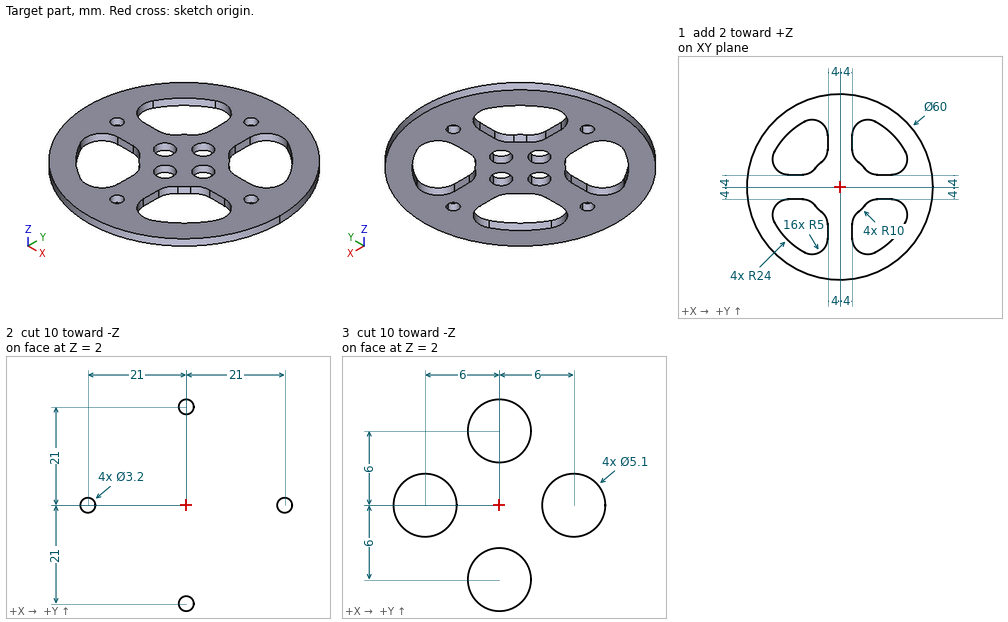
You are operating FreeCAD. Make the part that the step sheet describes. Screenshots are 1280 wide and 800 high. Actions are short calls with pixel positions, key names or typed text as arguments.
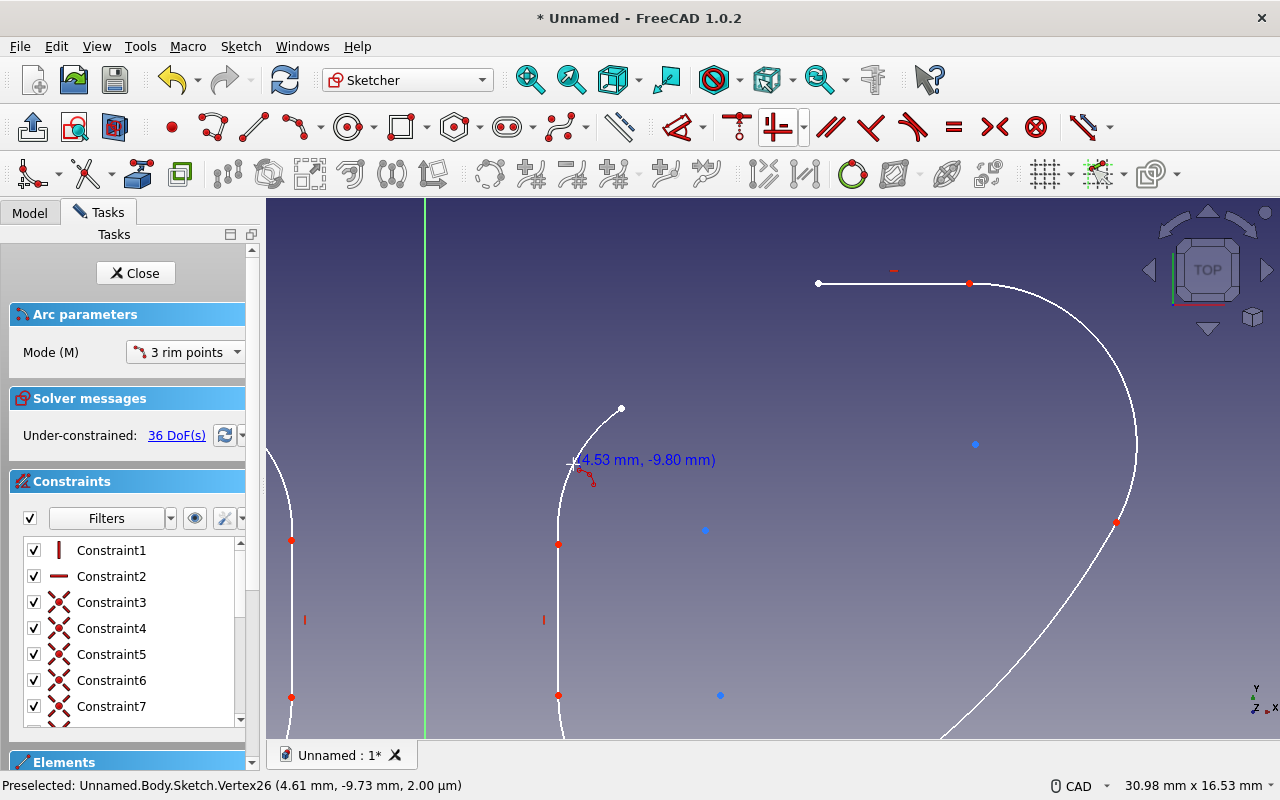
scroll(760, 533, down, 9)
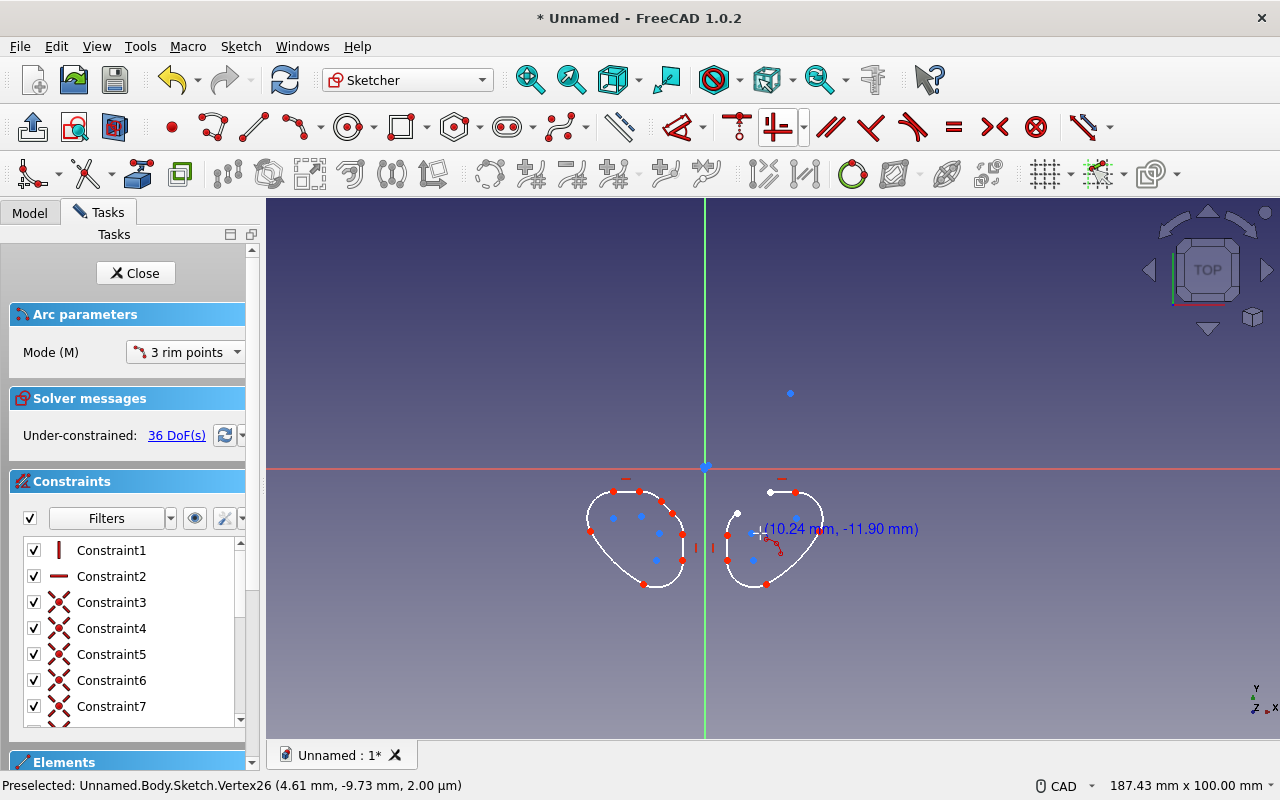
click(737, 513)
click(748, 502)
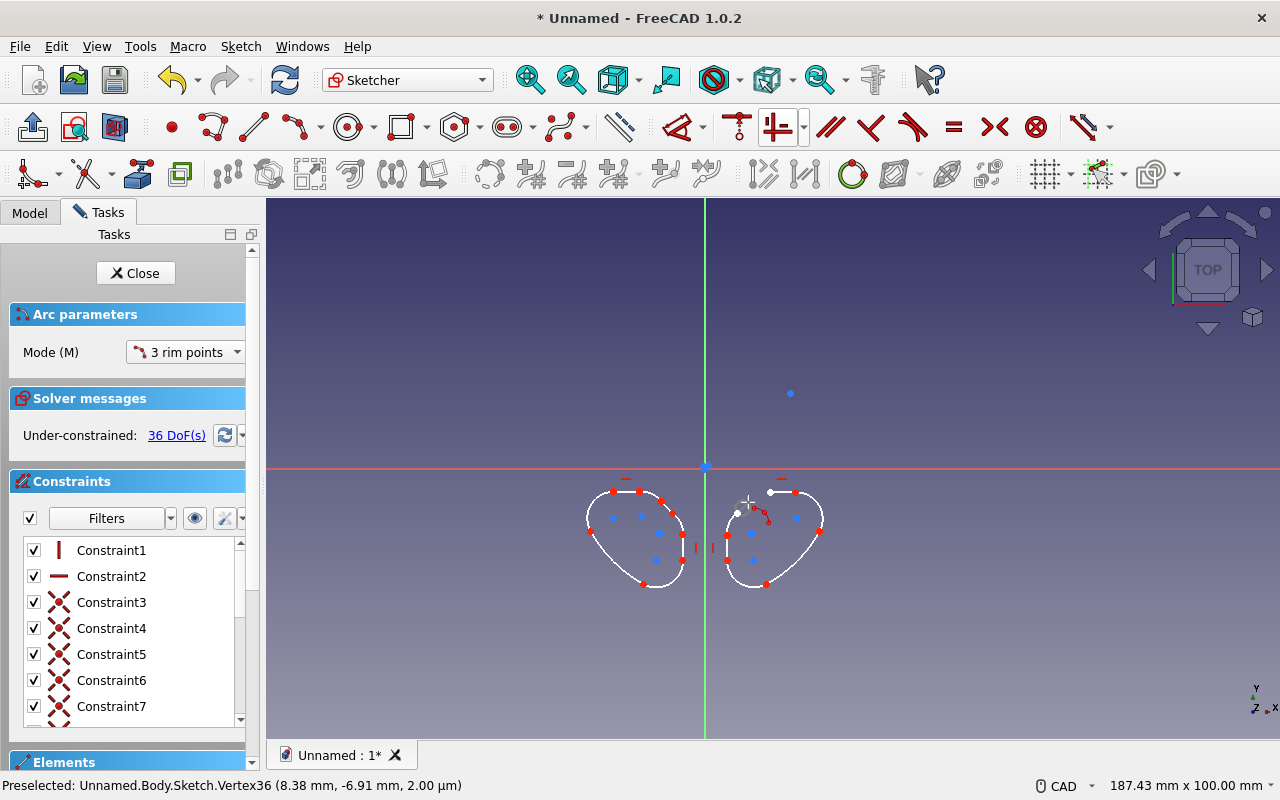
scroll(743, 508, up, 17)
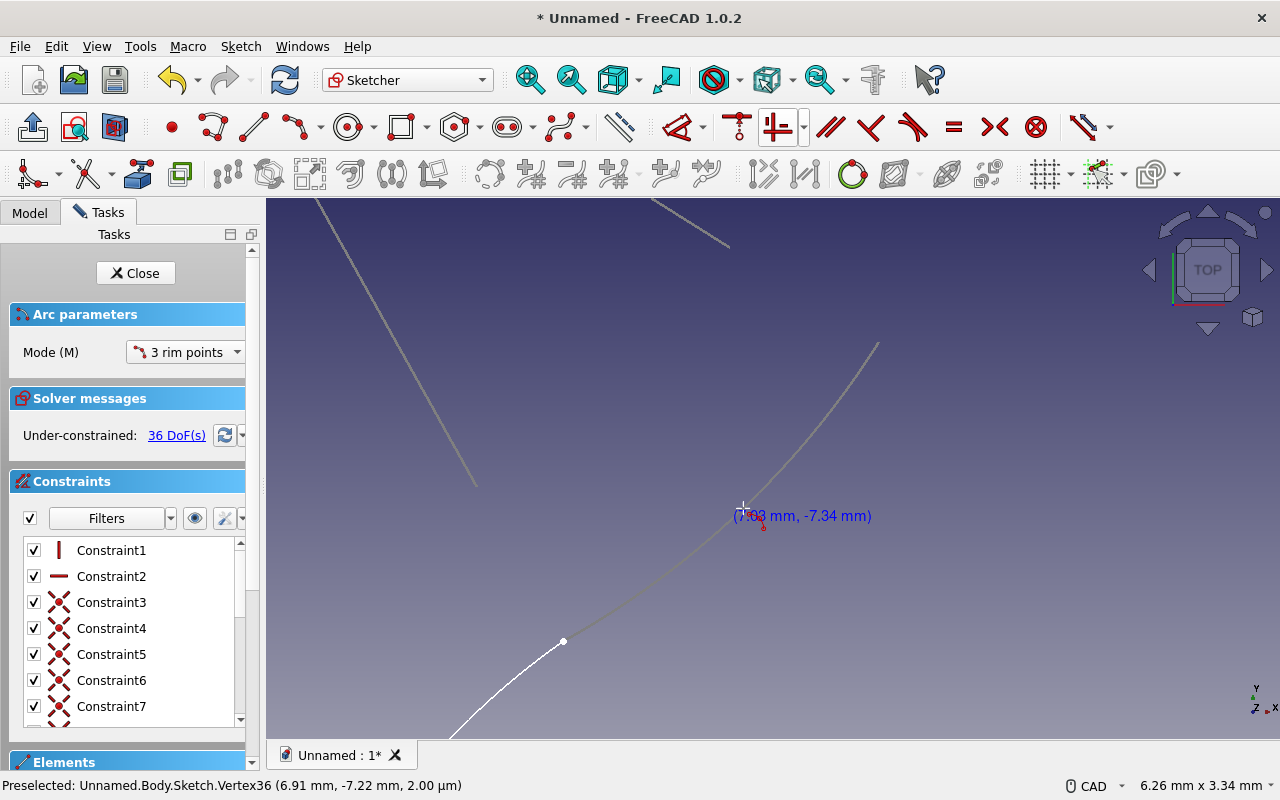
click(737, 478)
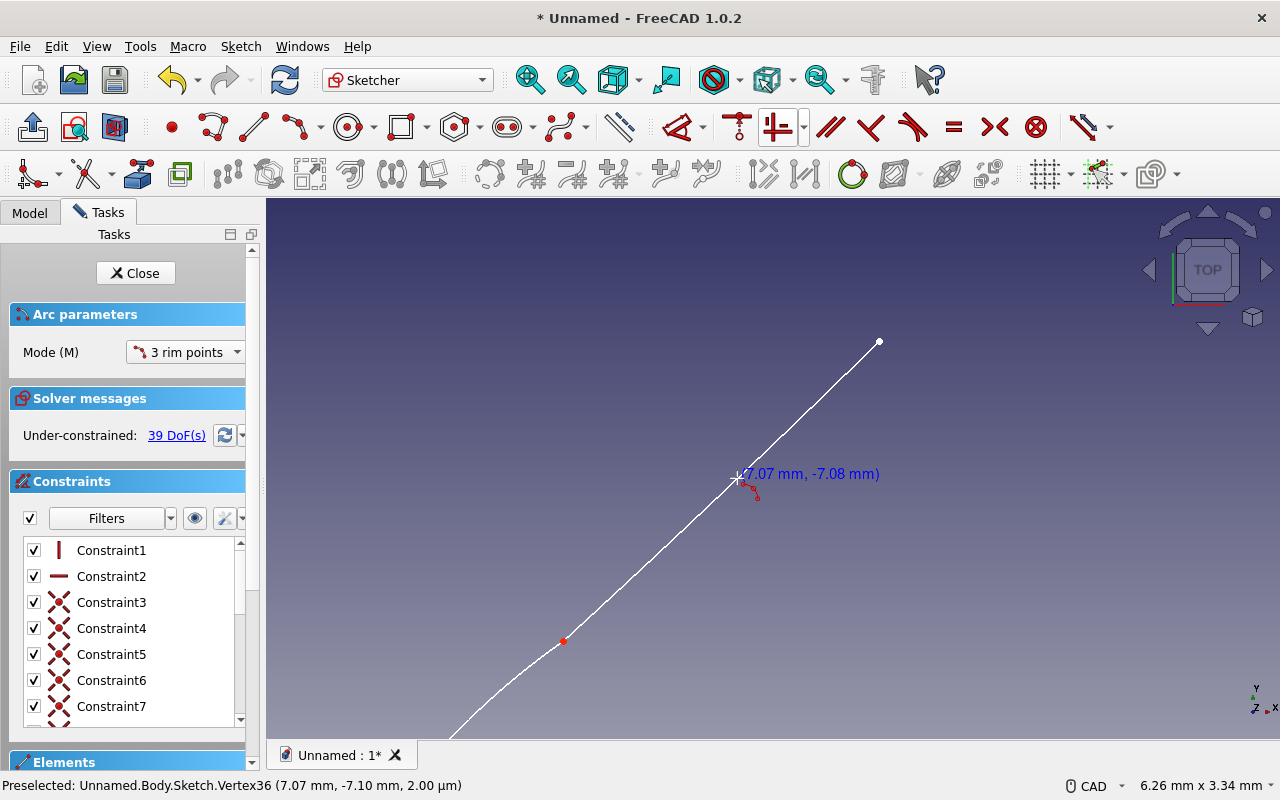
scroll(752, 517, down, 16)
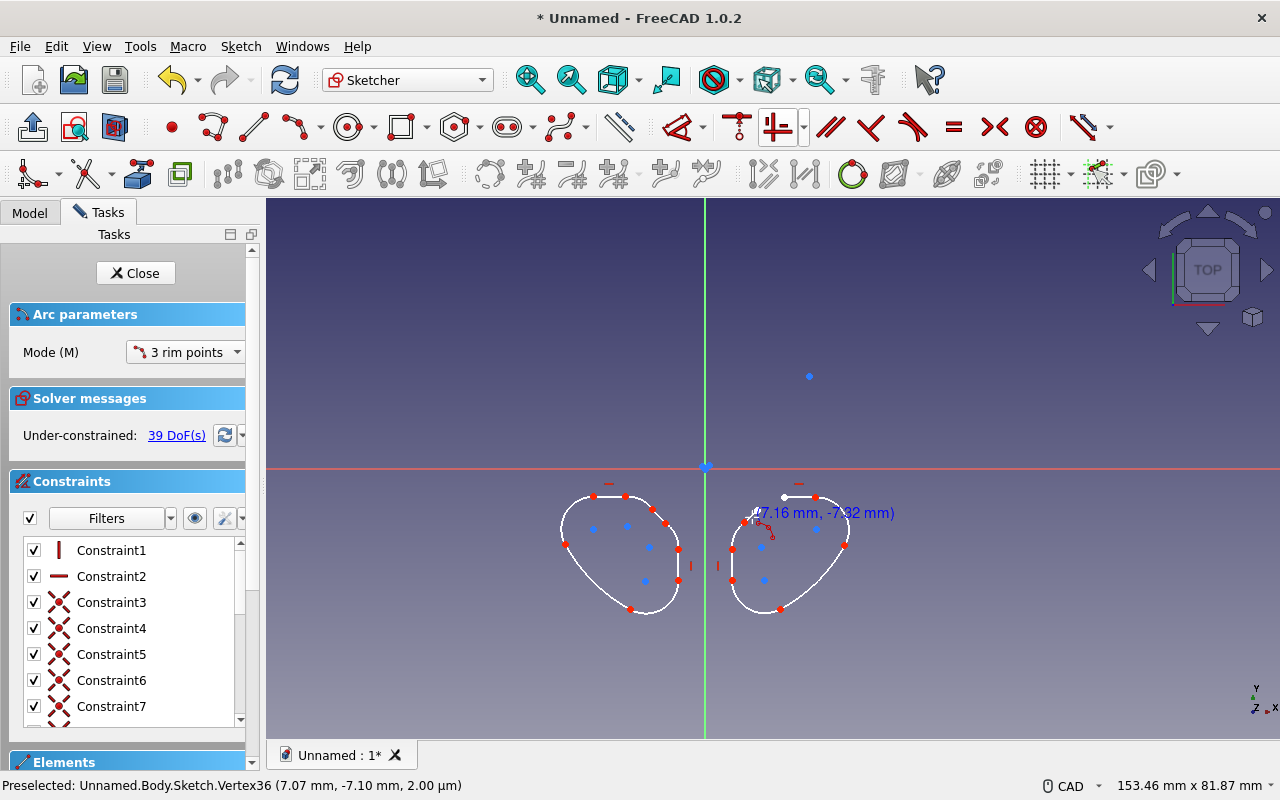
click(758, 510)
click(785, 497)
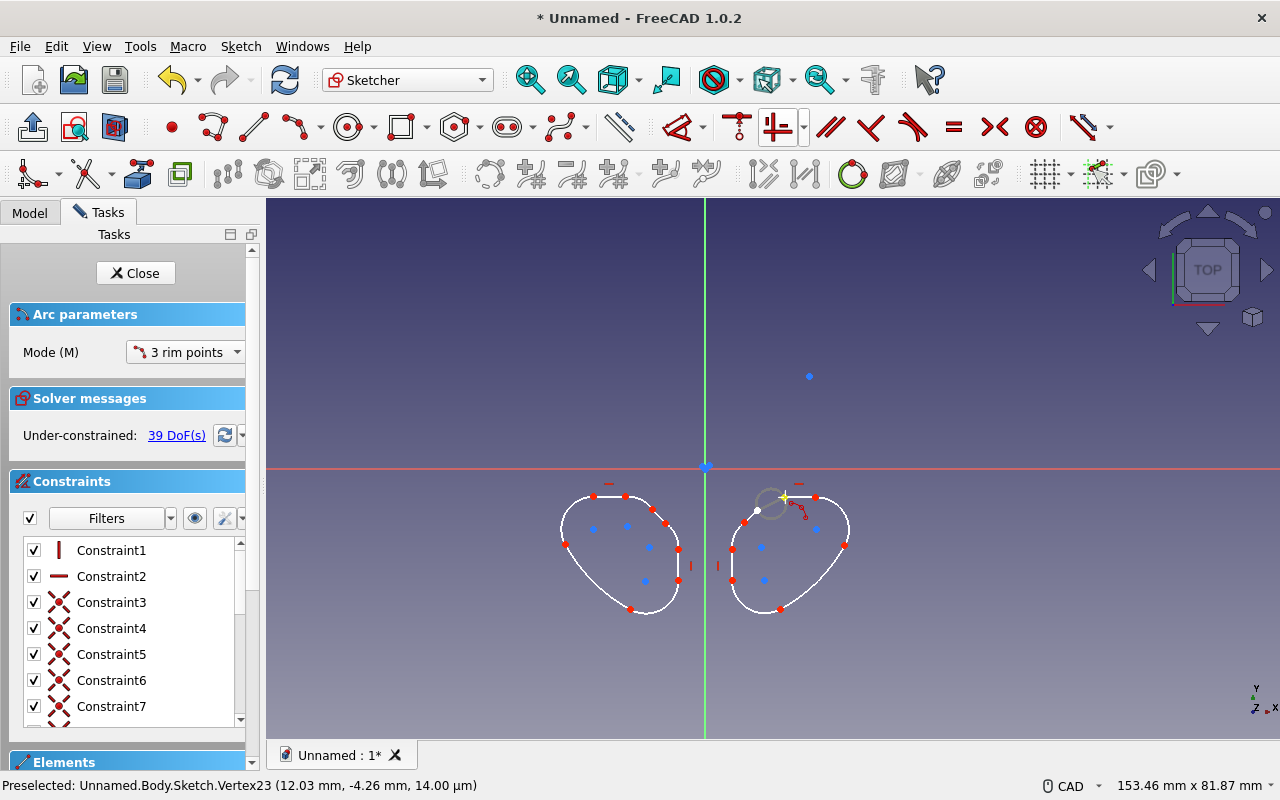
scroll(770, 499, up, 8)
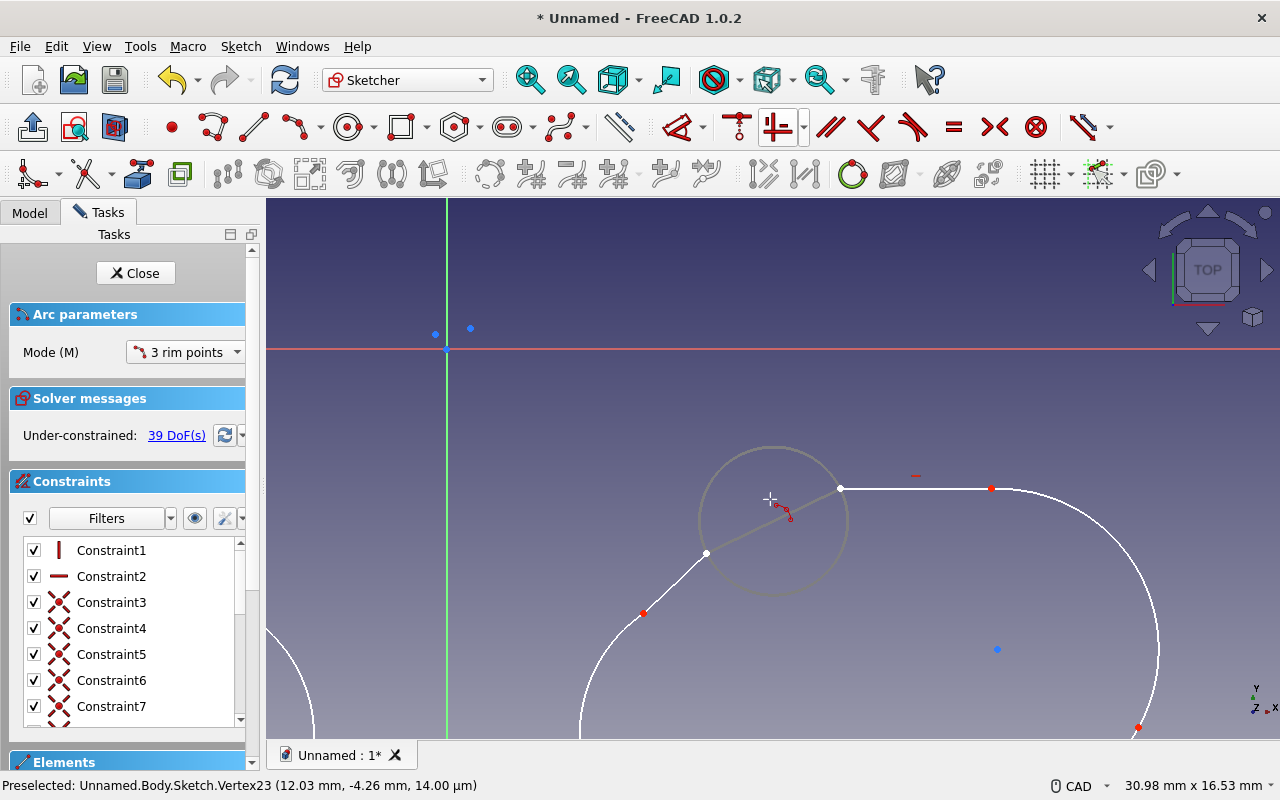
click(766, 498)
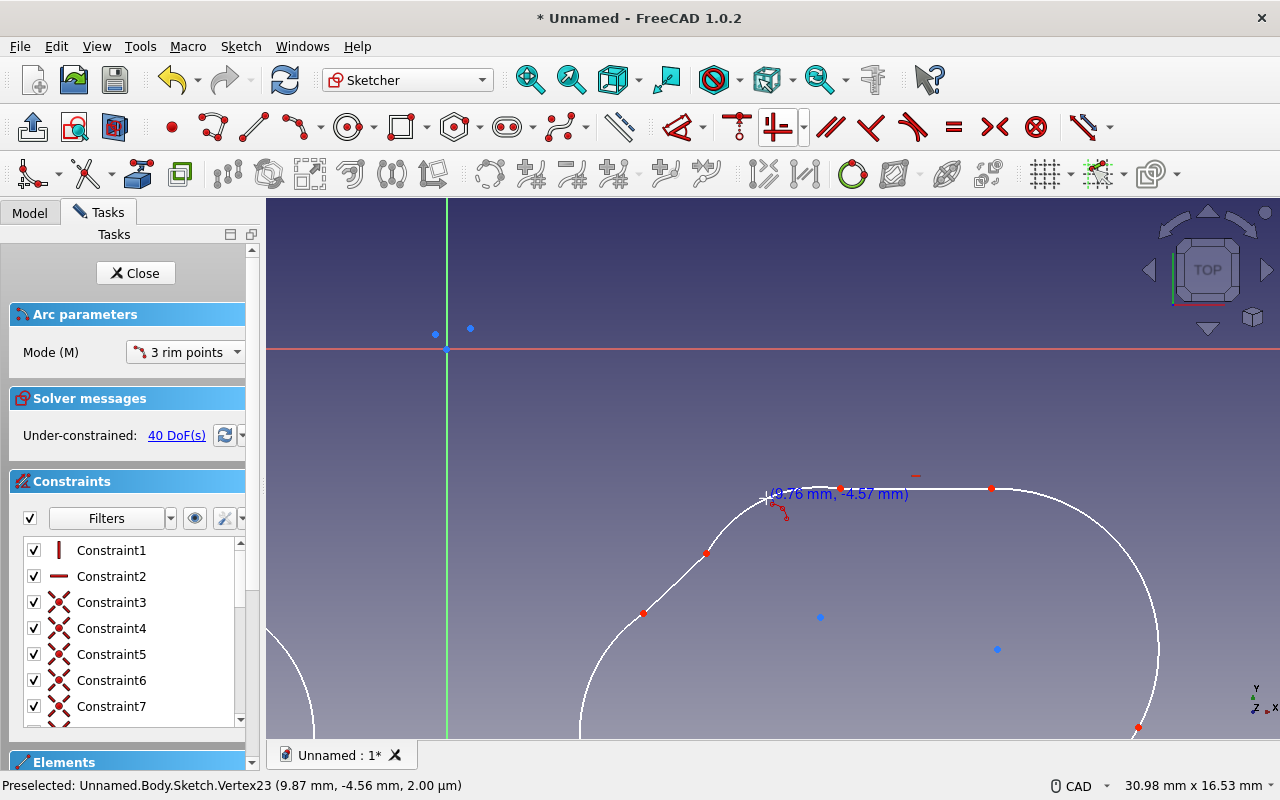
click(254, 128)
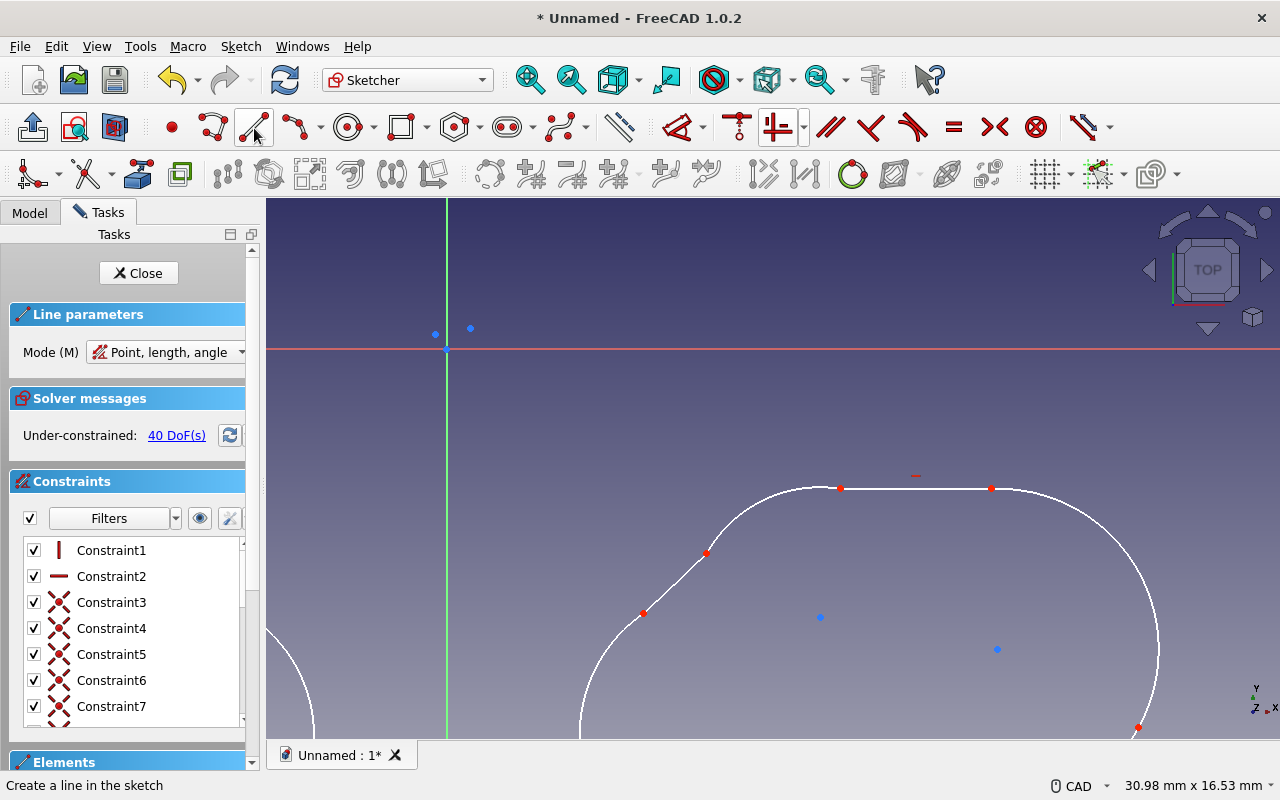
scroll(756, 492, down, 9)